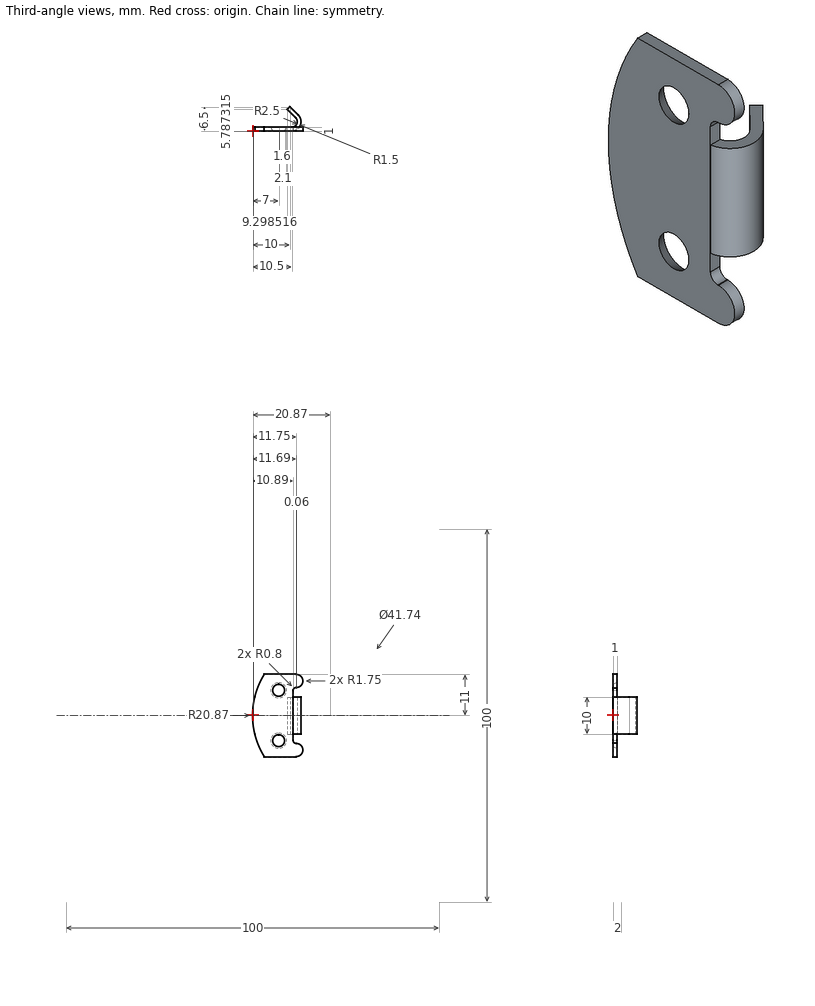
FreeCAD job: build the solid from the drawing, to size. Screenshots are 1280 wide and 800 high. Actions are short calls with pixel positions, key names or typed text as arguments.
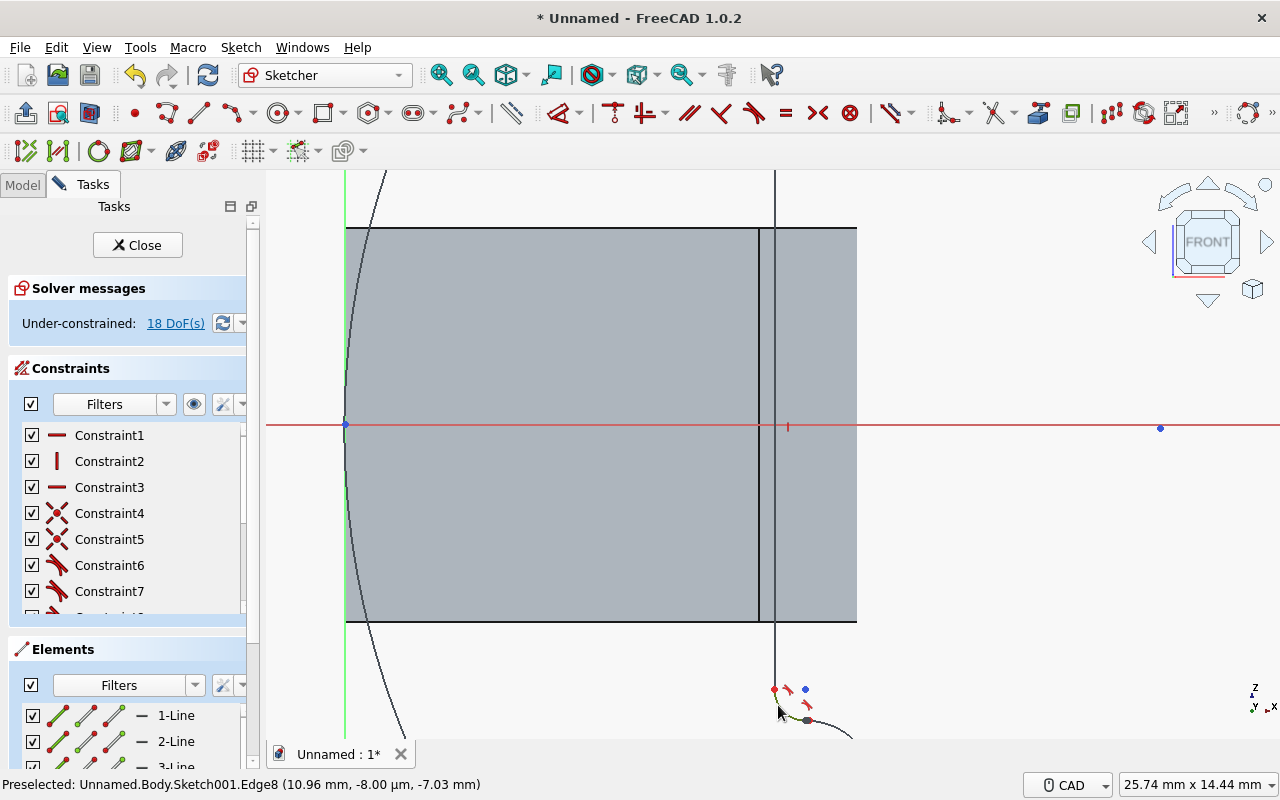
click(786, 114)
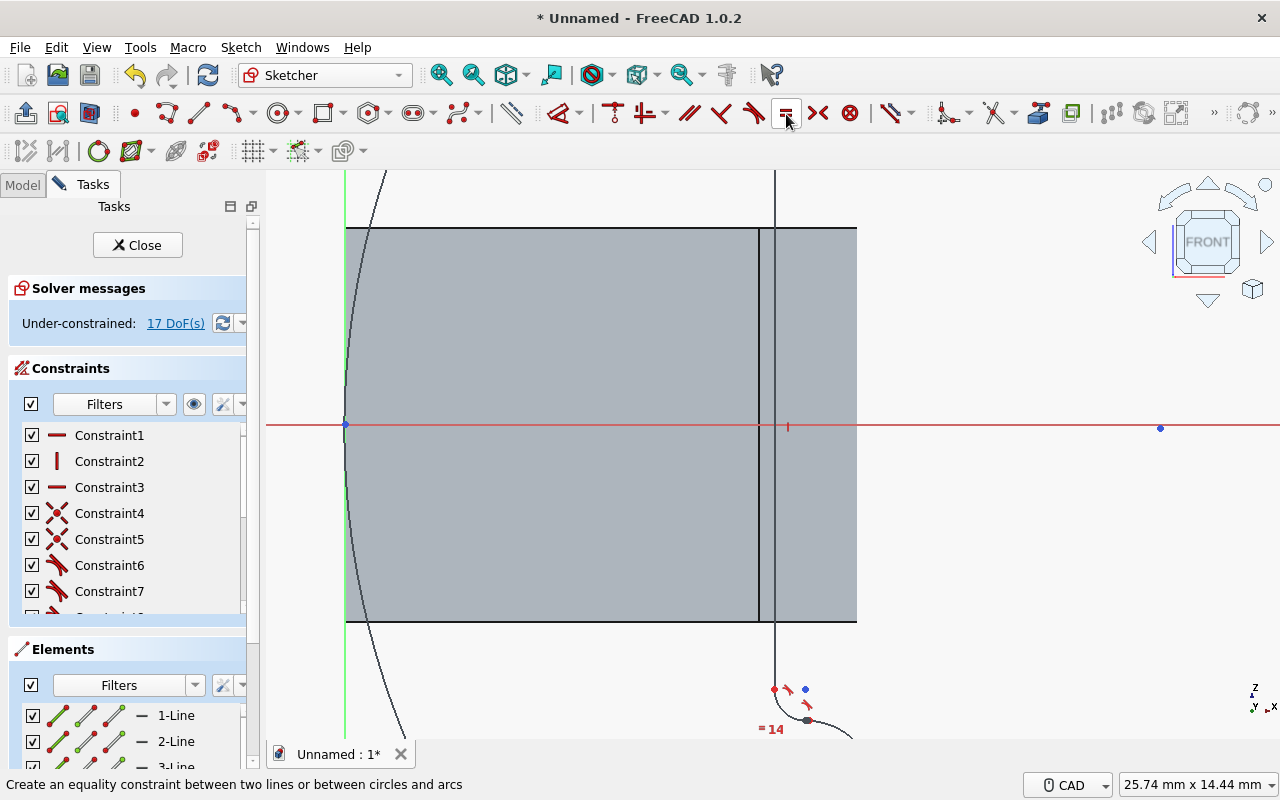
scroll(781, 479, down, 4)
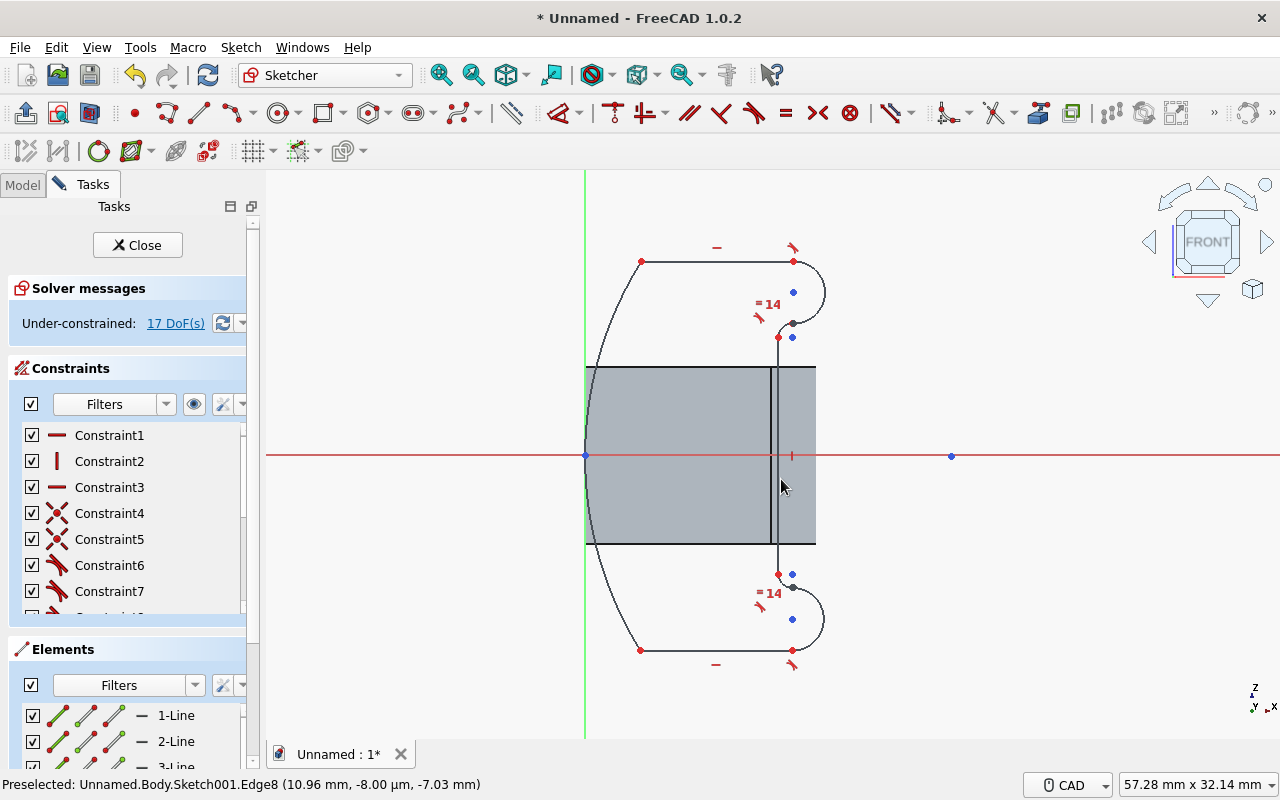
click(819, 311)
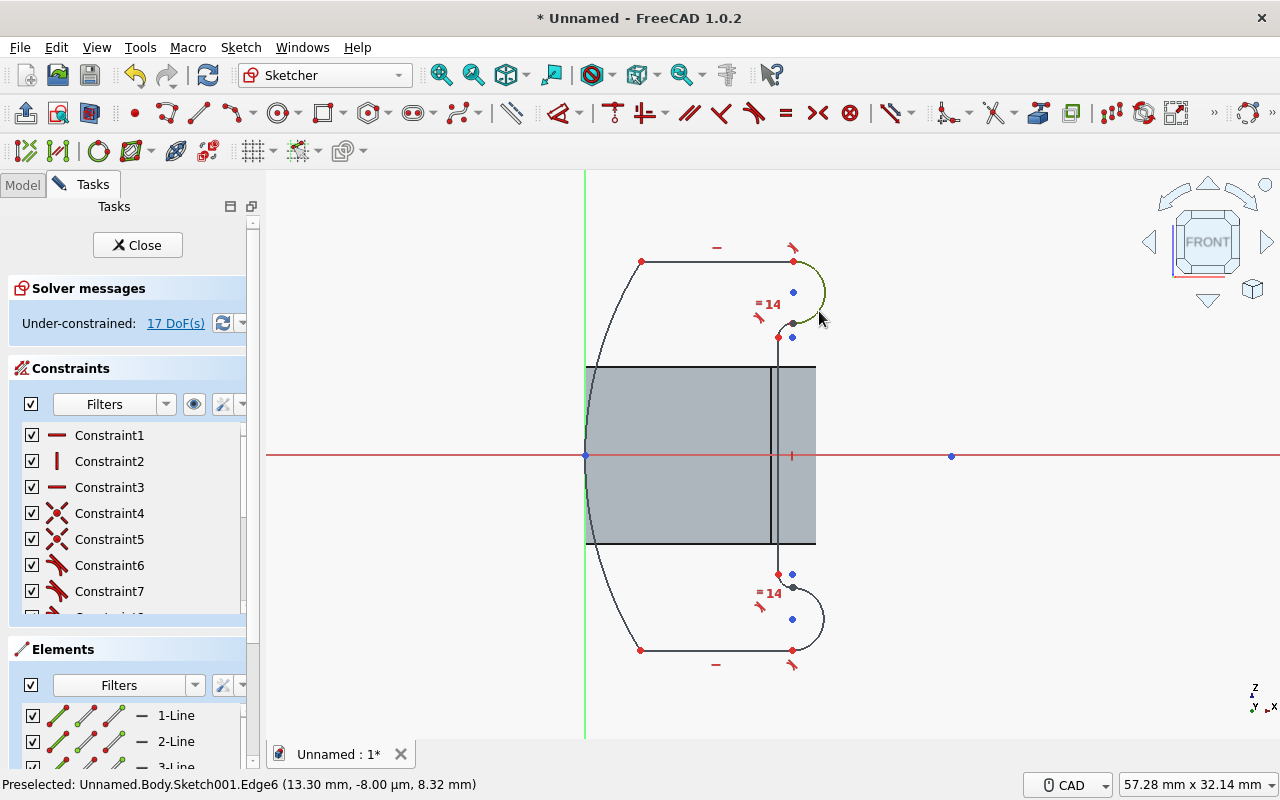
click(818, 638)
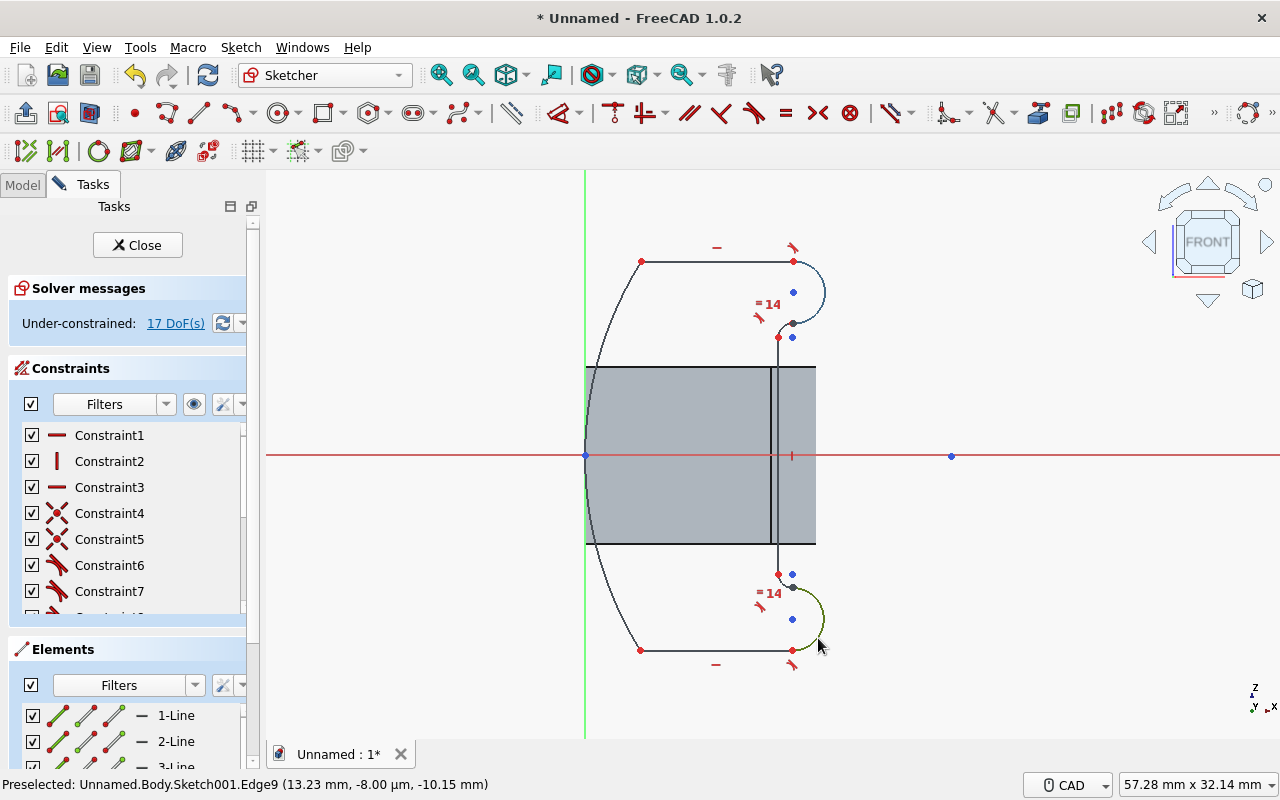
click(786, 114)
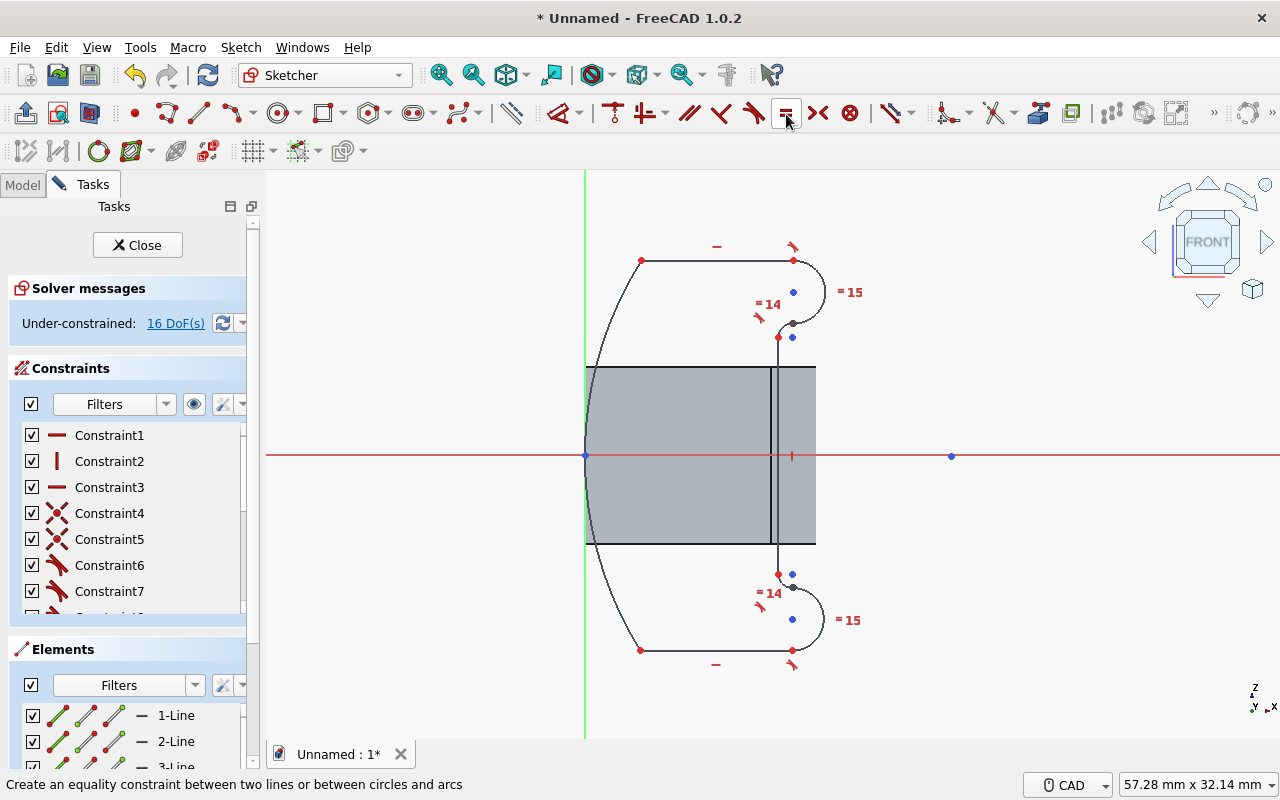
click(952, 456)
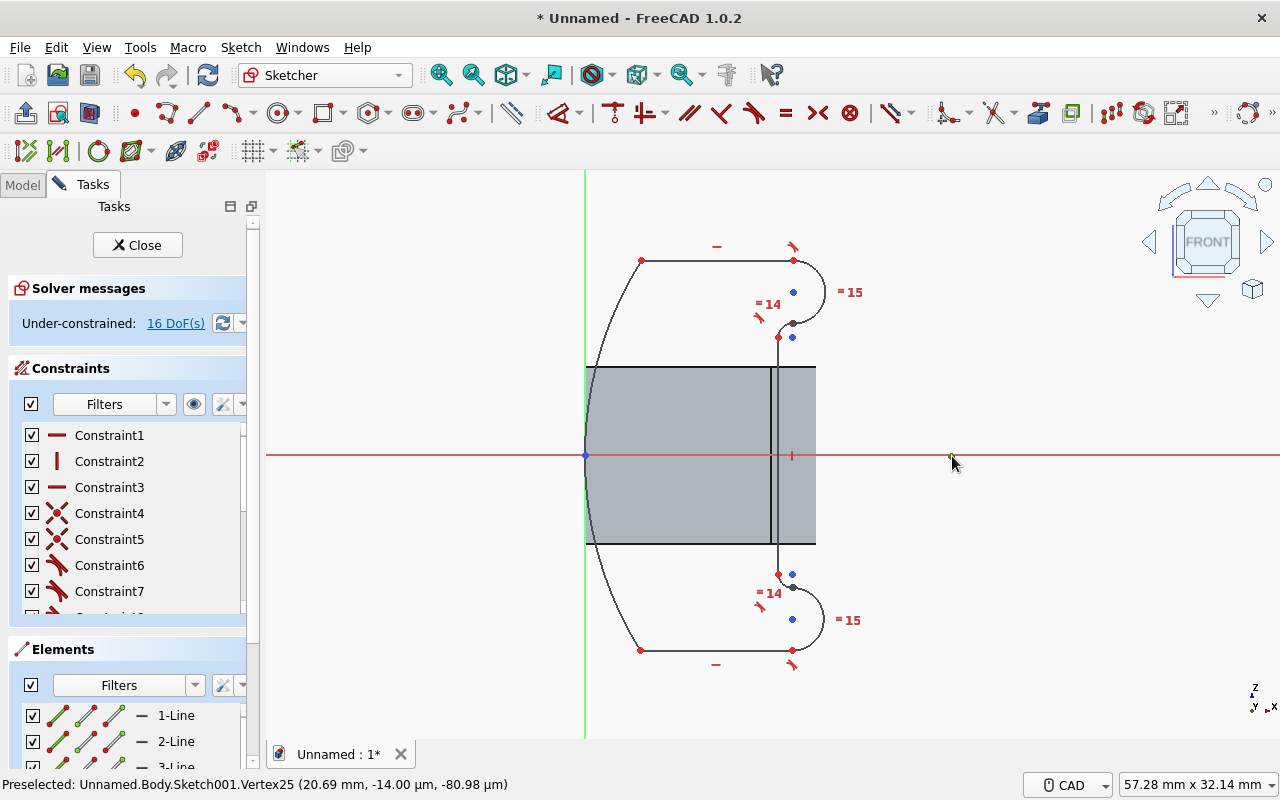
click(353, 455)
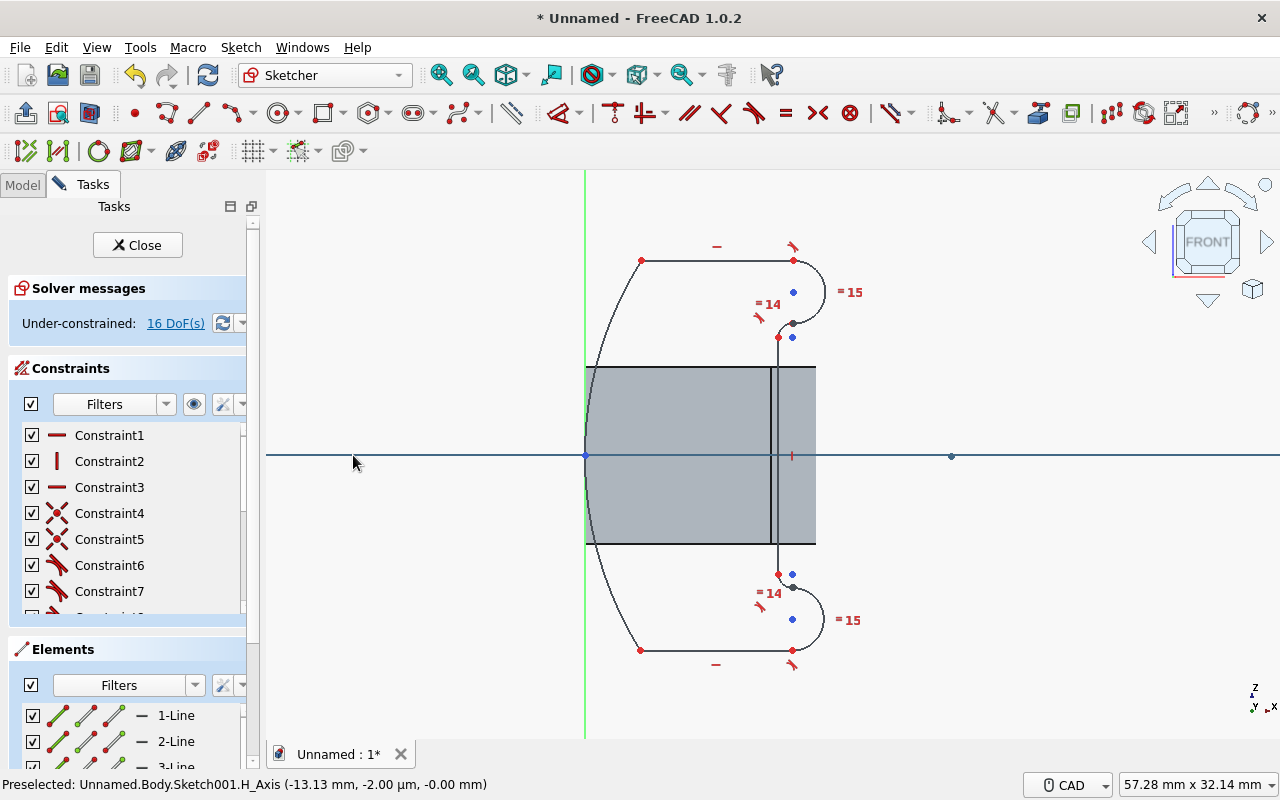
click(614, 114)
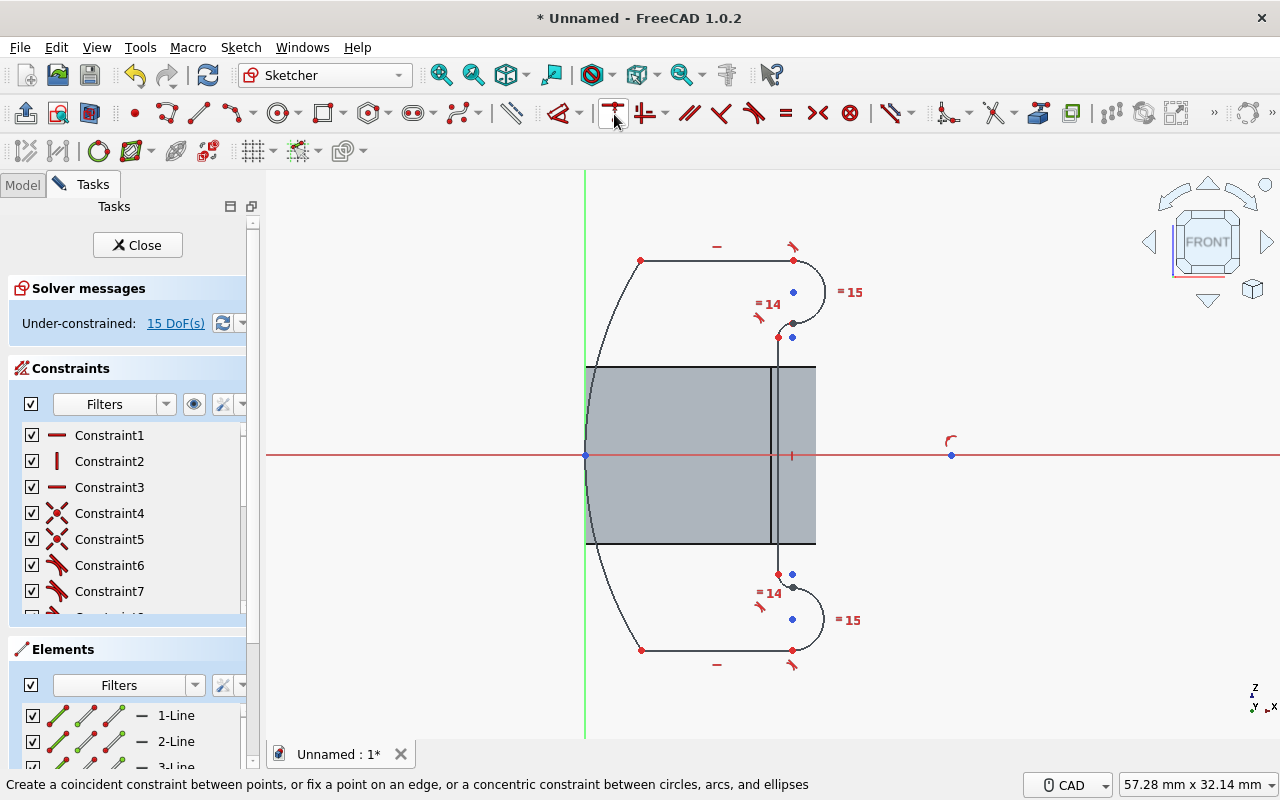
click(794, 292)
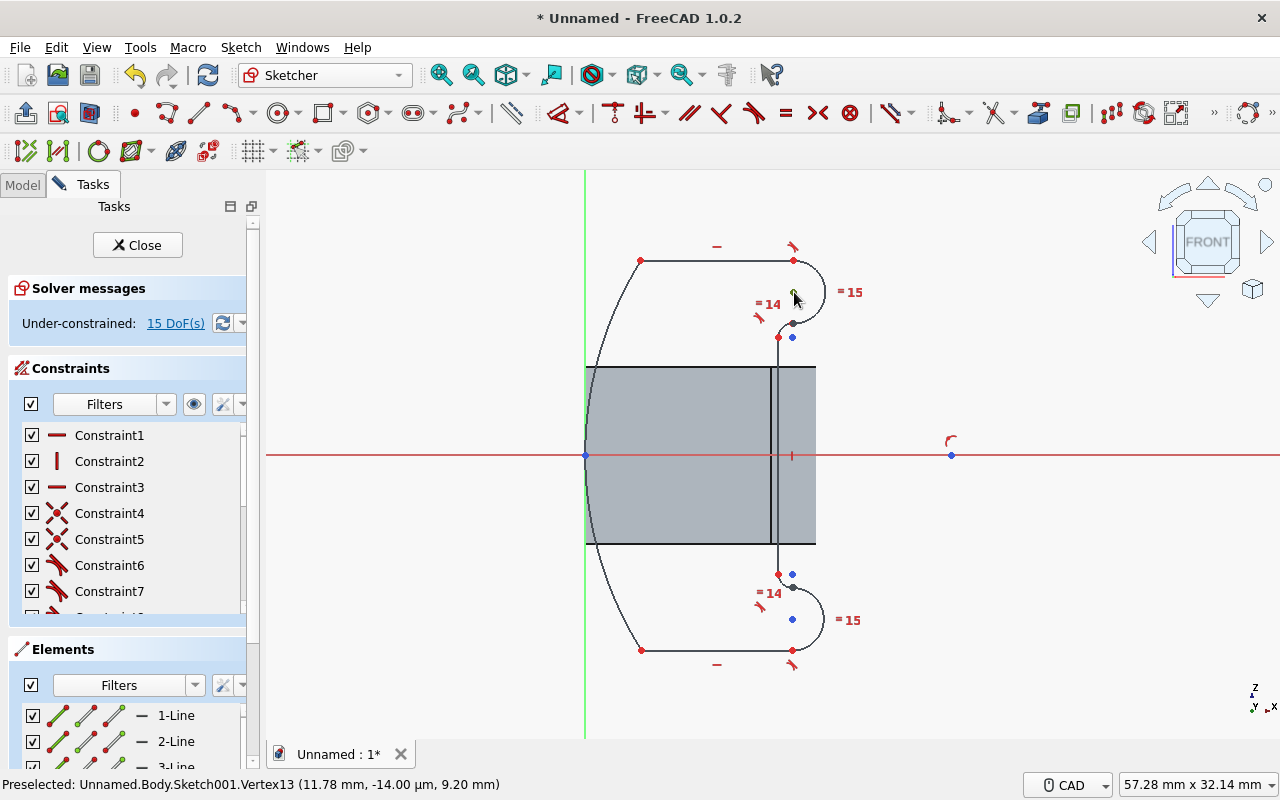
click(792, 619)